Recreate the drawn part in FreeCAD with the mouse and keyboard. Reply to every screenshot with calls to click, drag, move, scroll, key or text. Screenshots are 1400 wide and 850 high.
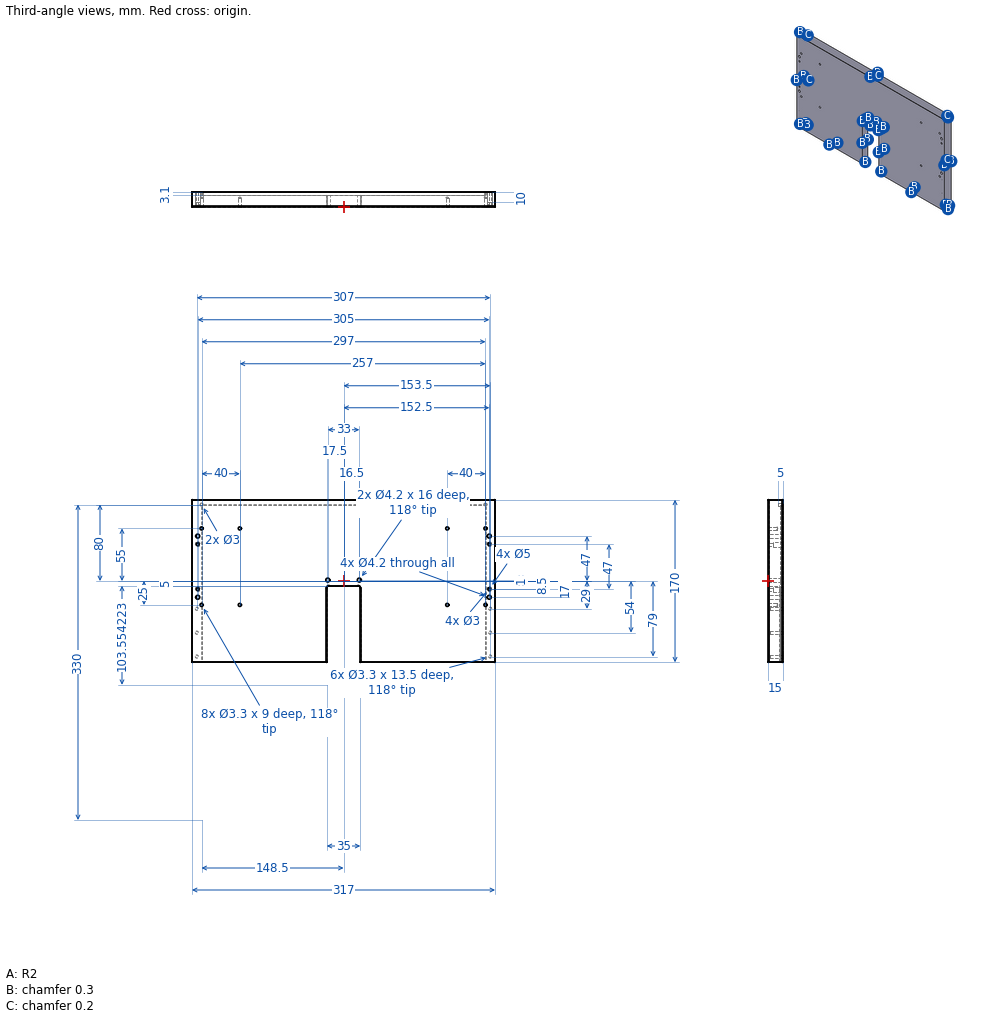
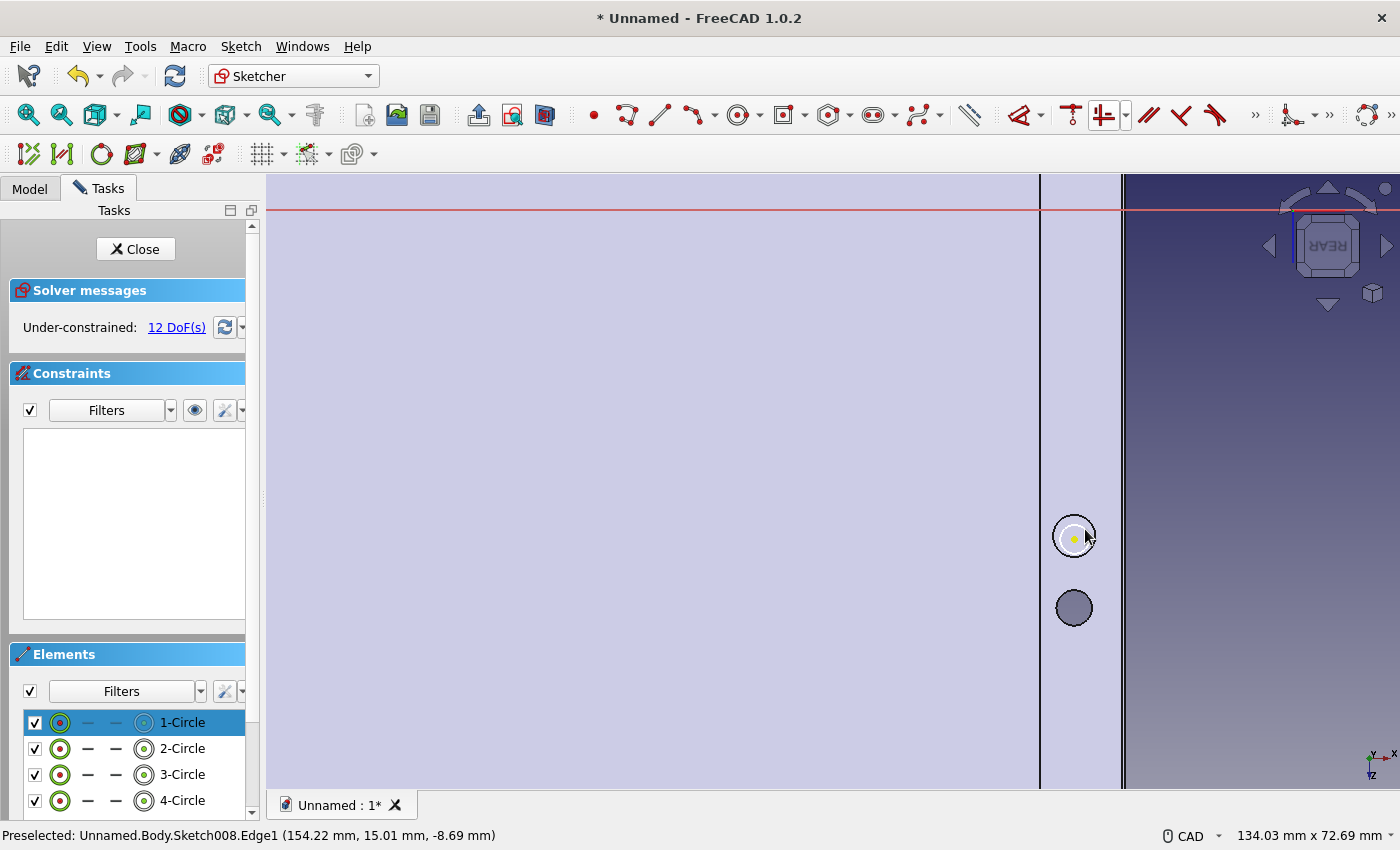
click(1085, 529)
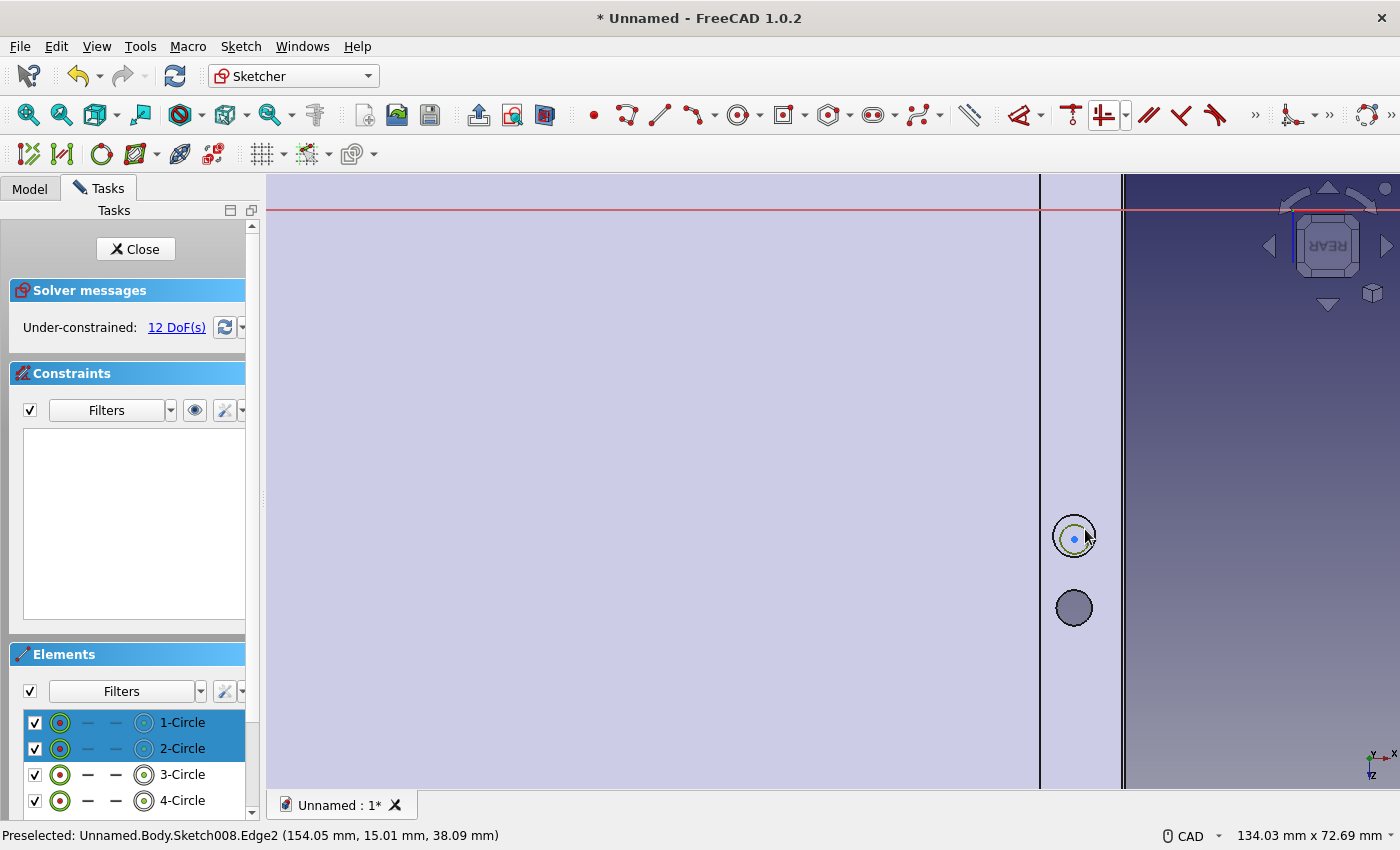
scroll(1085, 529, down, 7)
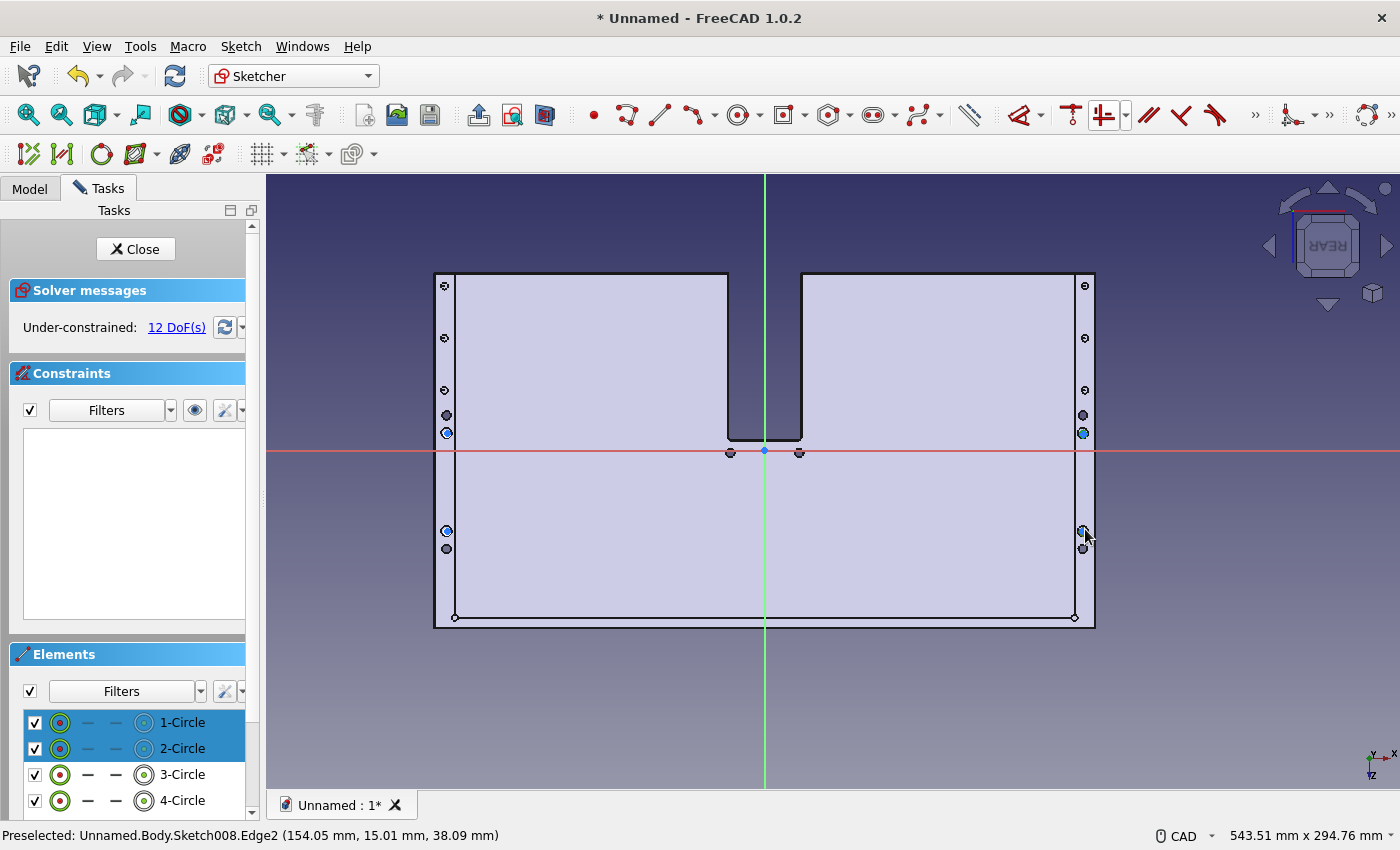
scroll(449, 432, up, 7)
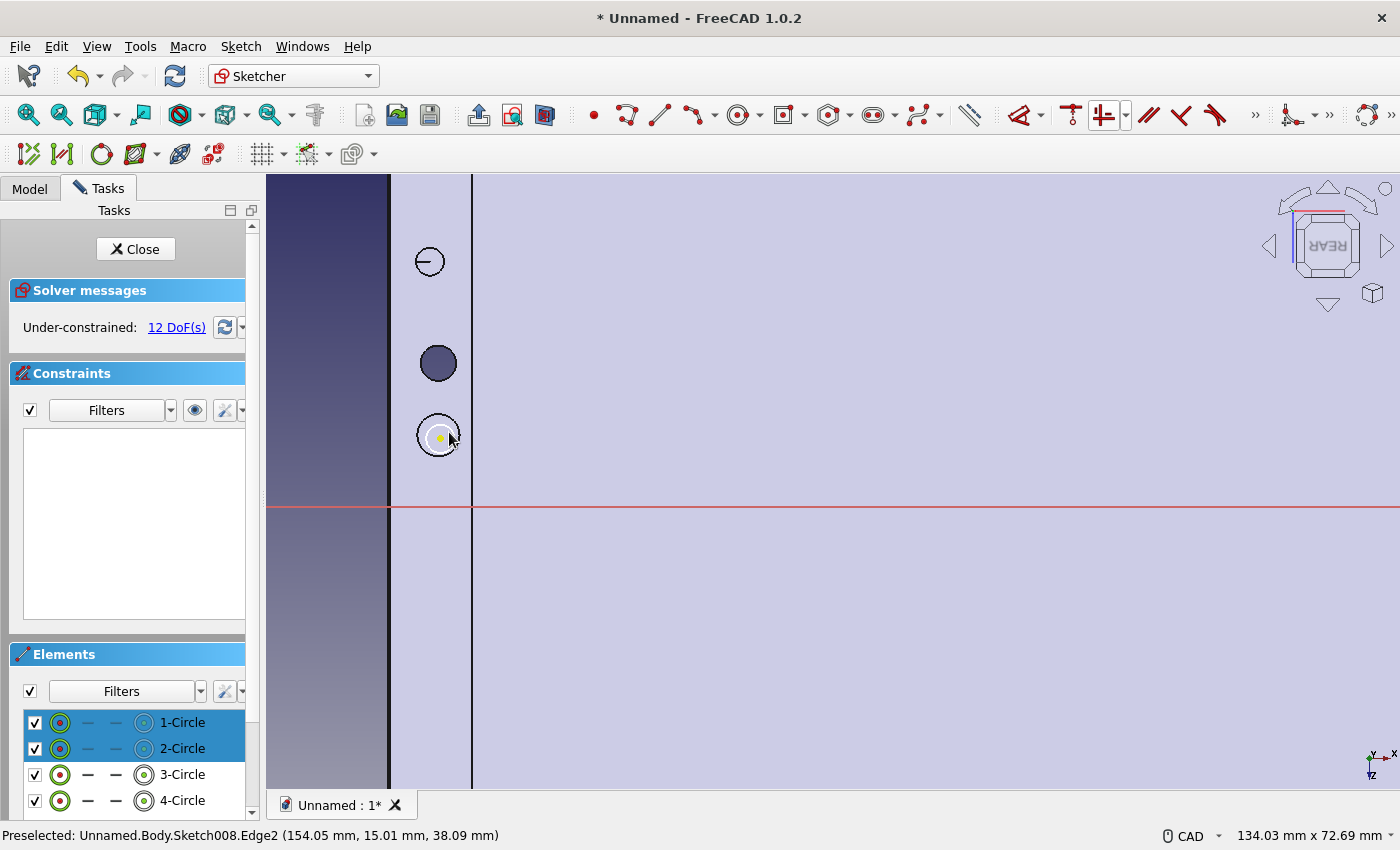
click(450, 429)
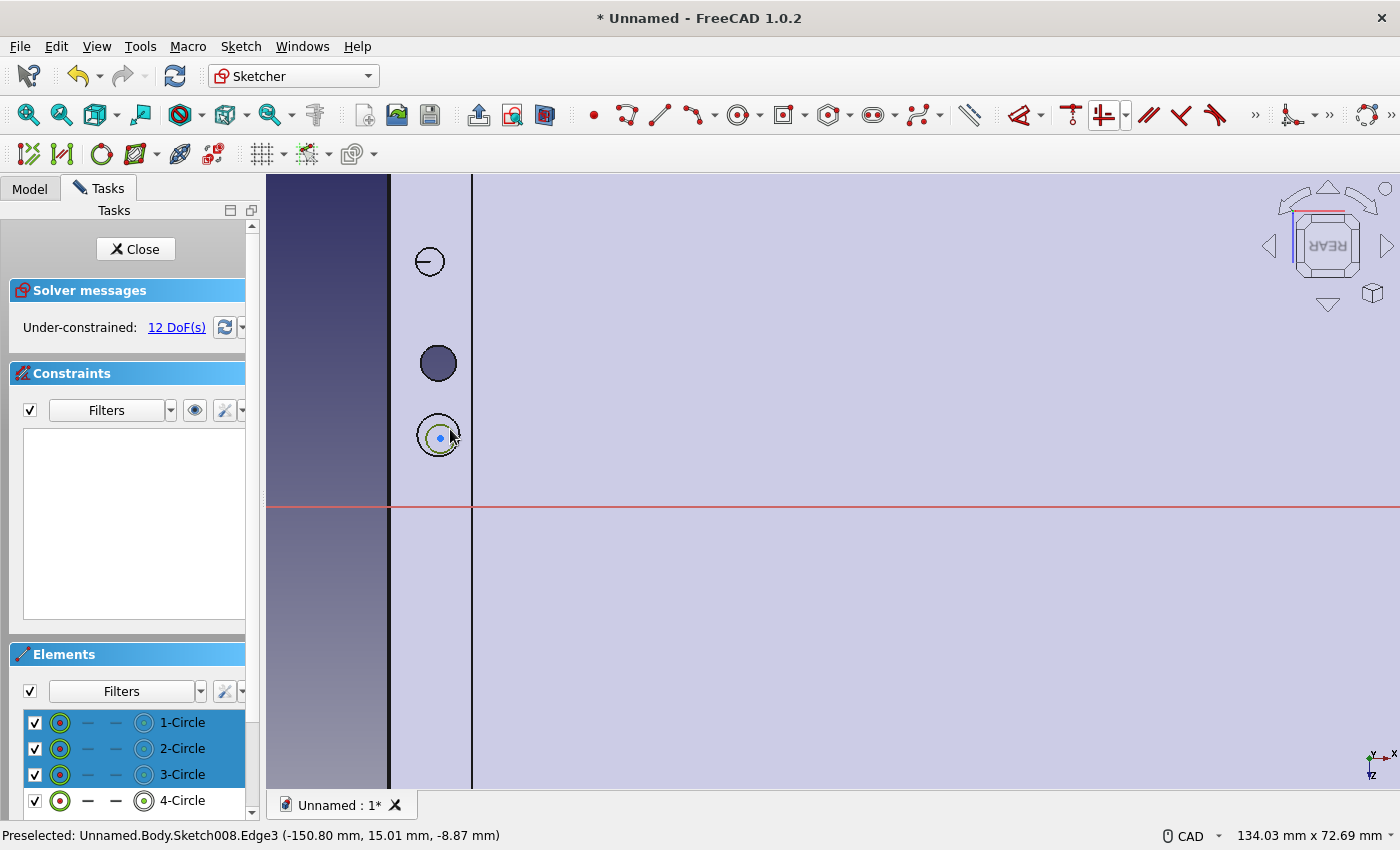
scroll(449, 432, down, 7)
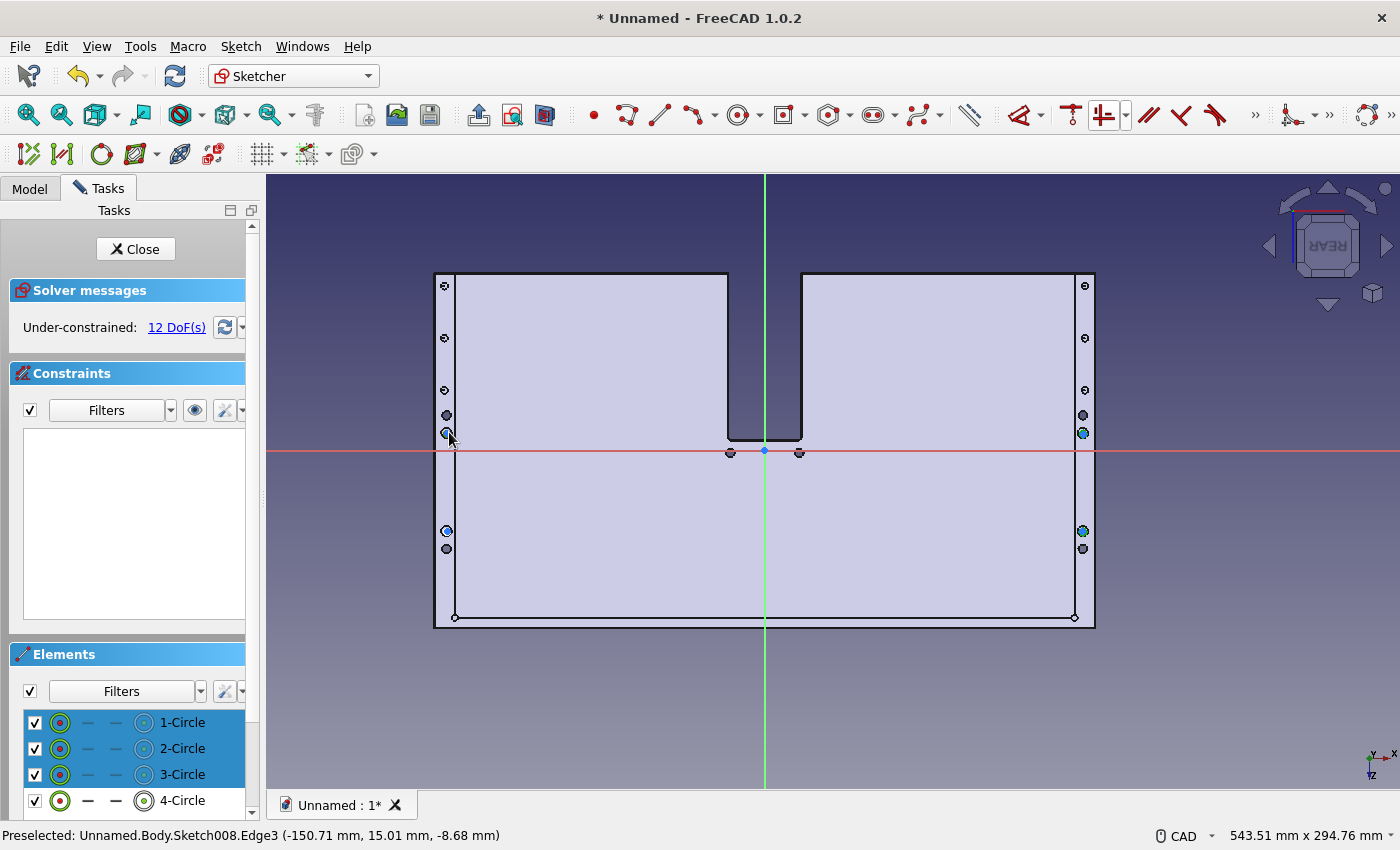
scroll(449, 530, up, 8)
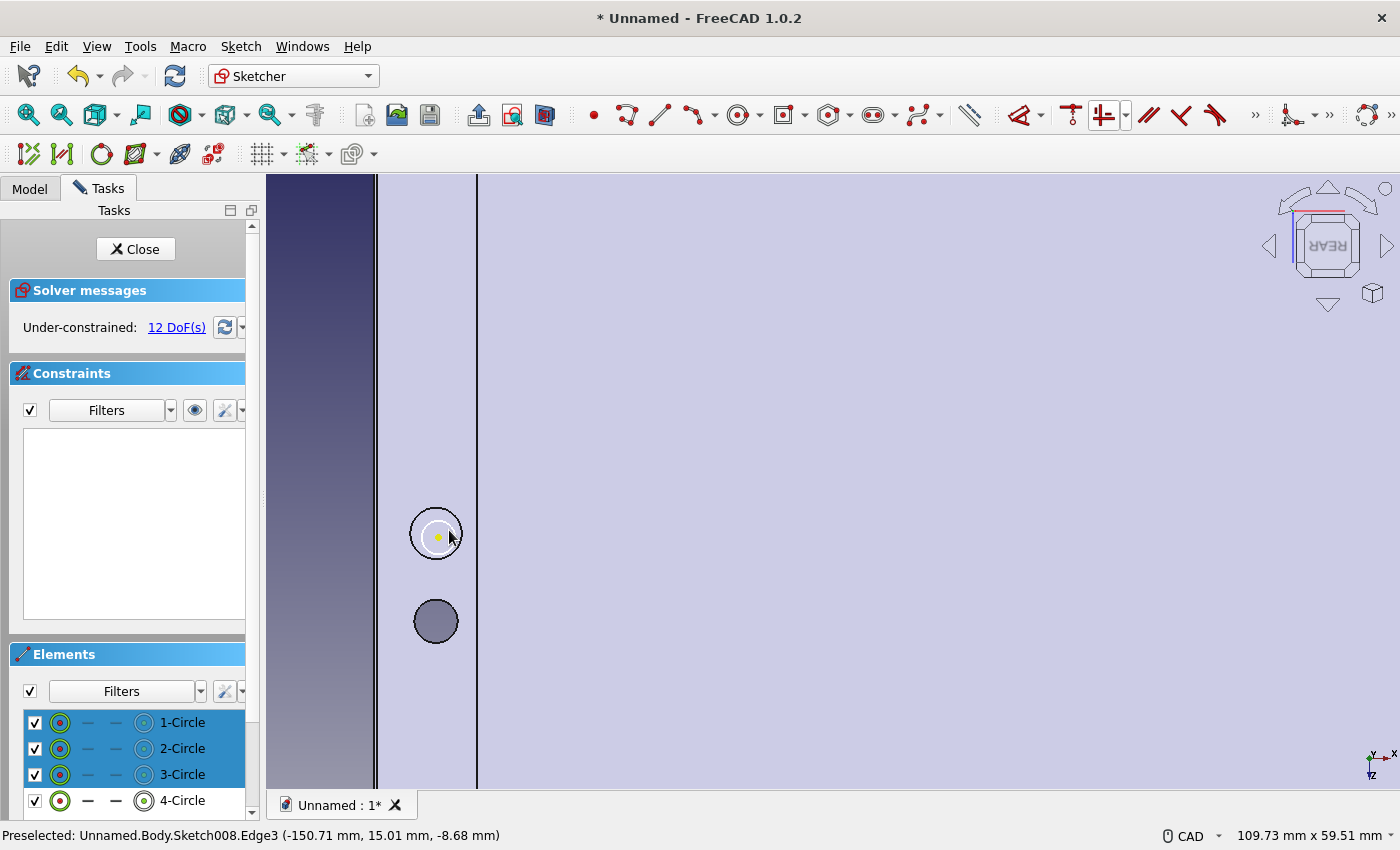
click(450, 526)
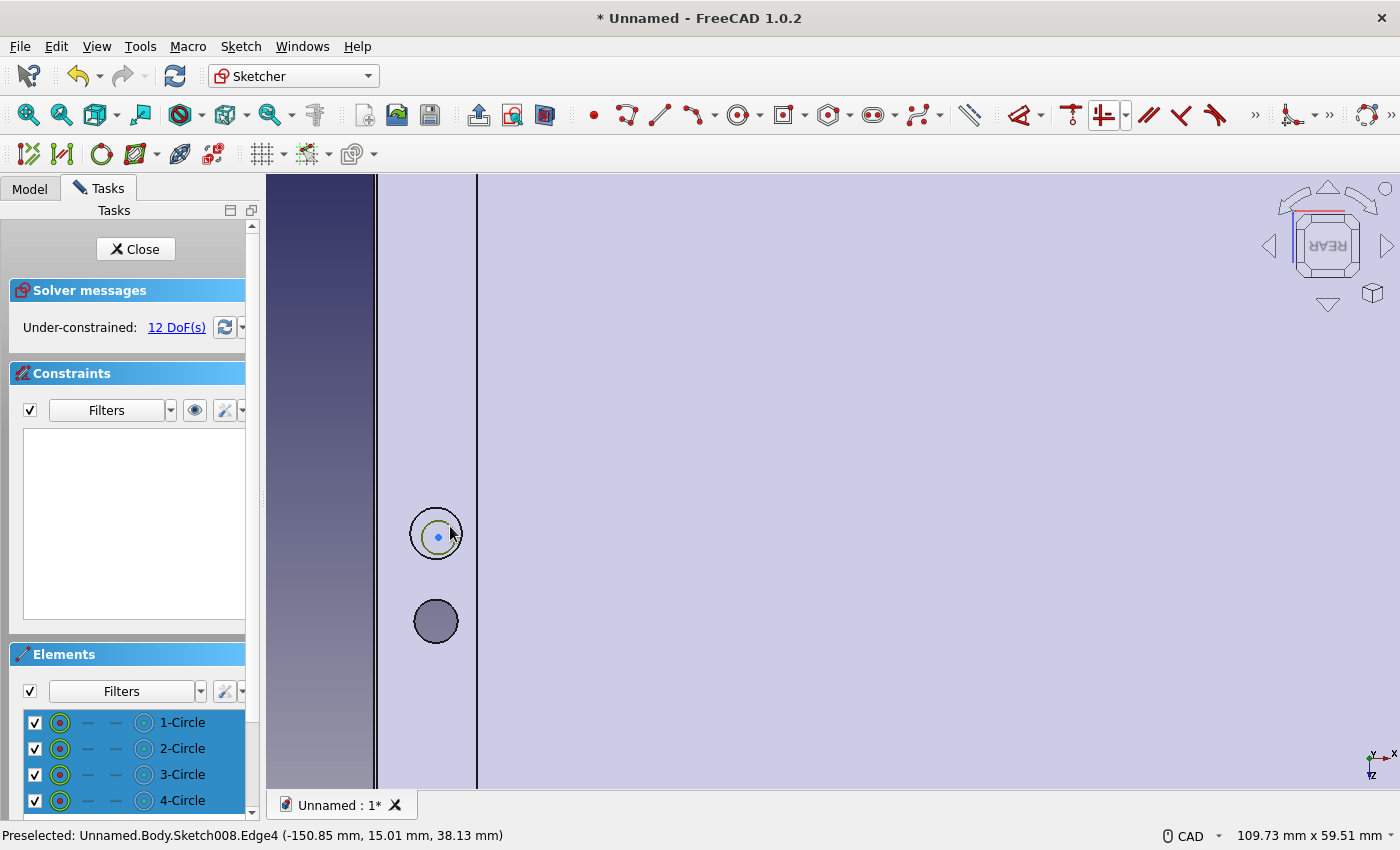
key(e)